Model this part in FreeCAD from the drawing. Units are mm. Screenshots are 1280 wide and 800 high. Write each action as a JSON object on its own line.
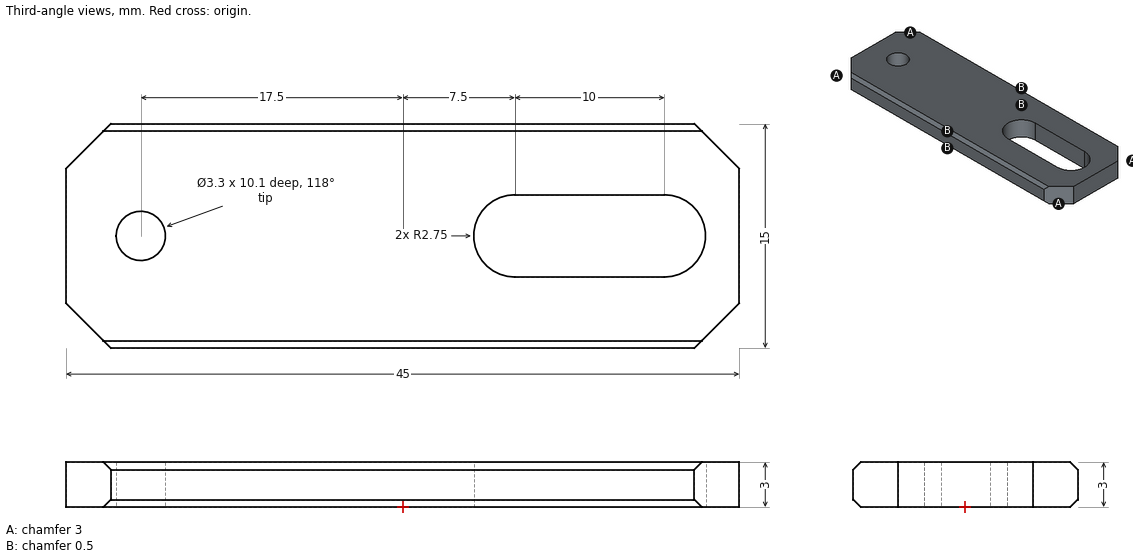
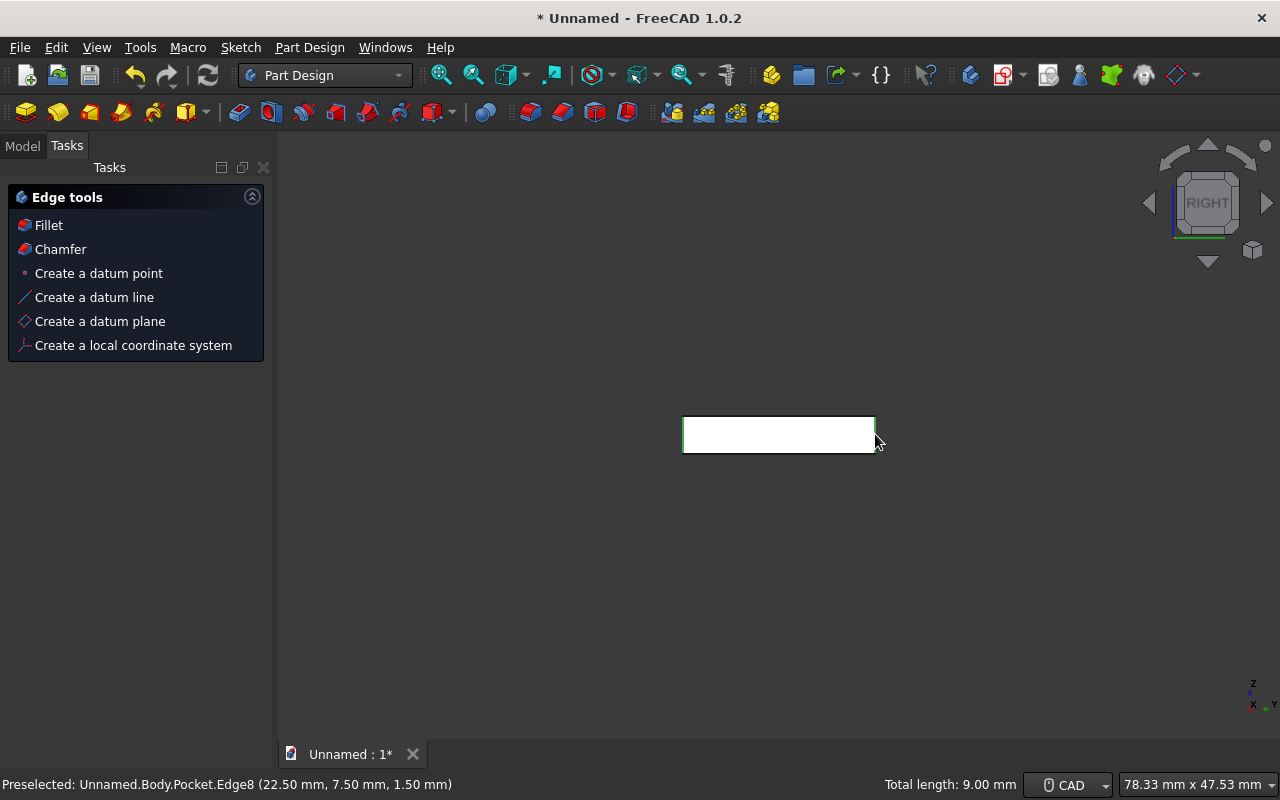
{"action": "key", "text": "5"}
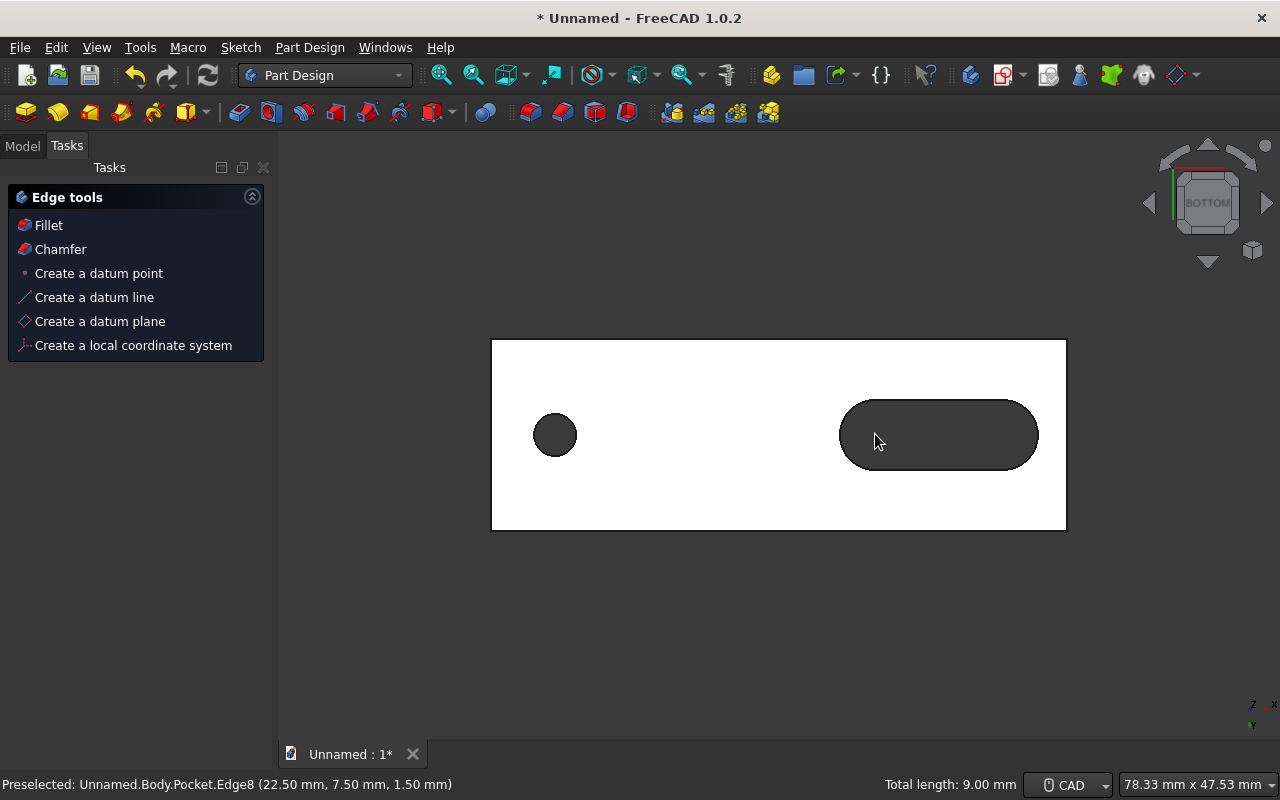
{"action": "key", "text": "4"}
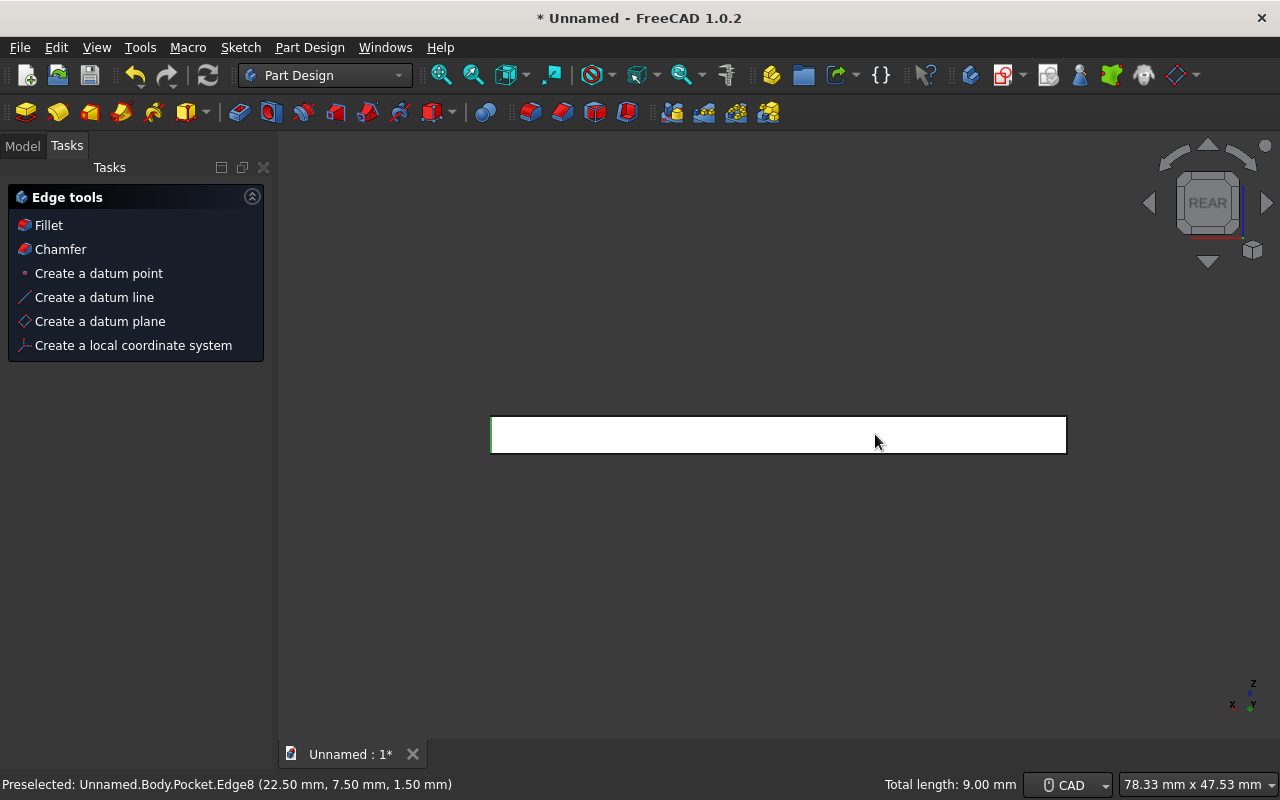
{"action": "left_click", "coordinate": [1067, 434], "text": "ctrl"}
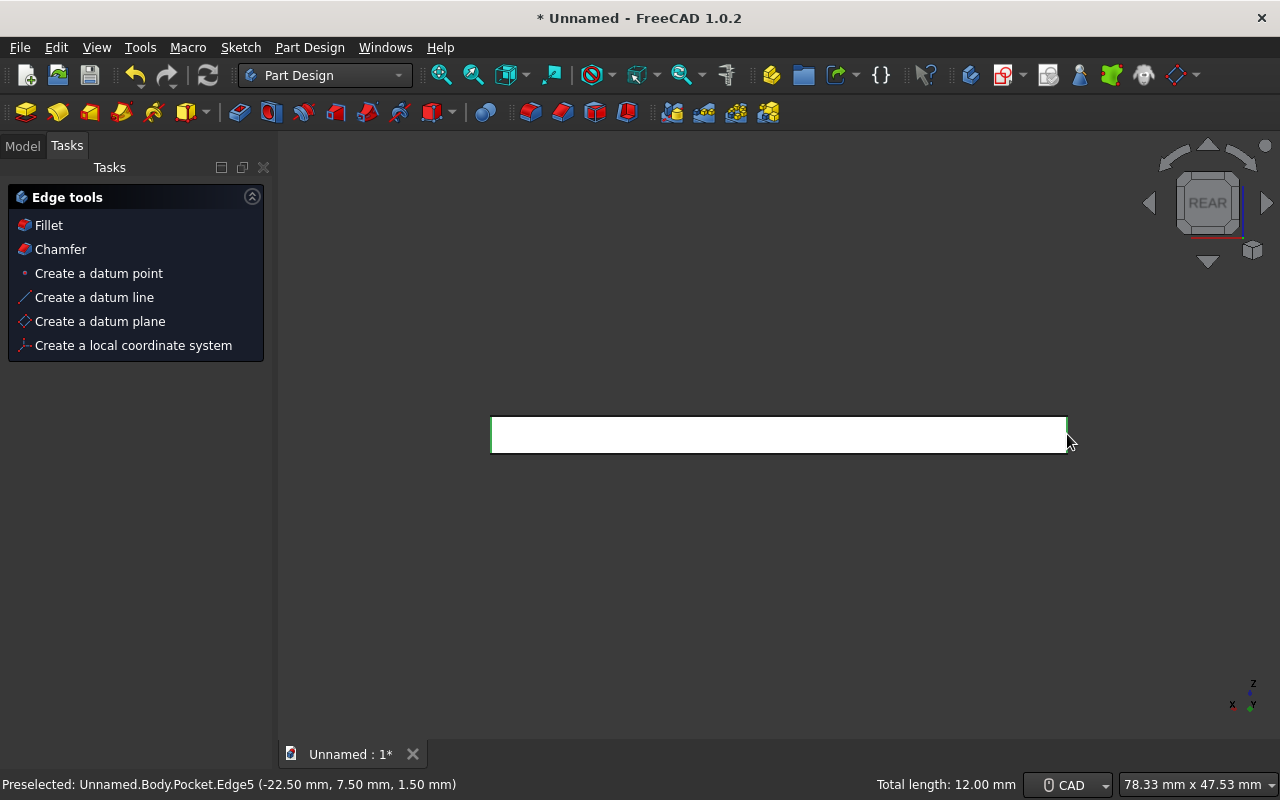
{"action": "left_click", "coordinate": [564, 112]}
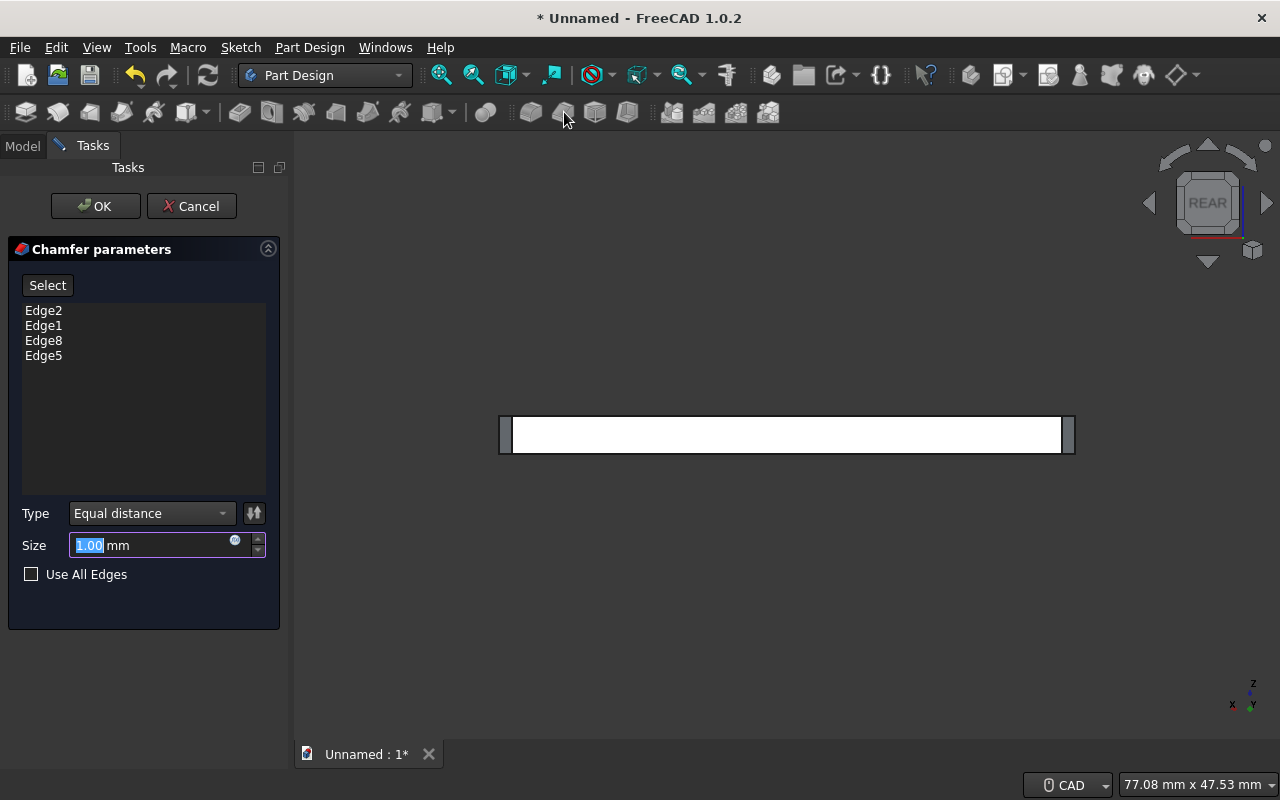
{"action": "type", "text": "3"}
{"action": "key", "text": "Tab"}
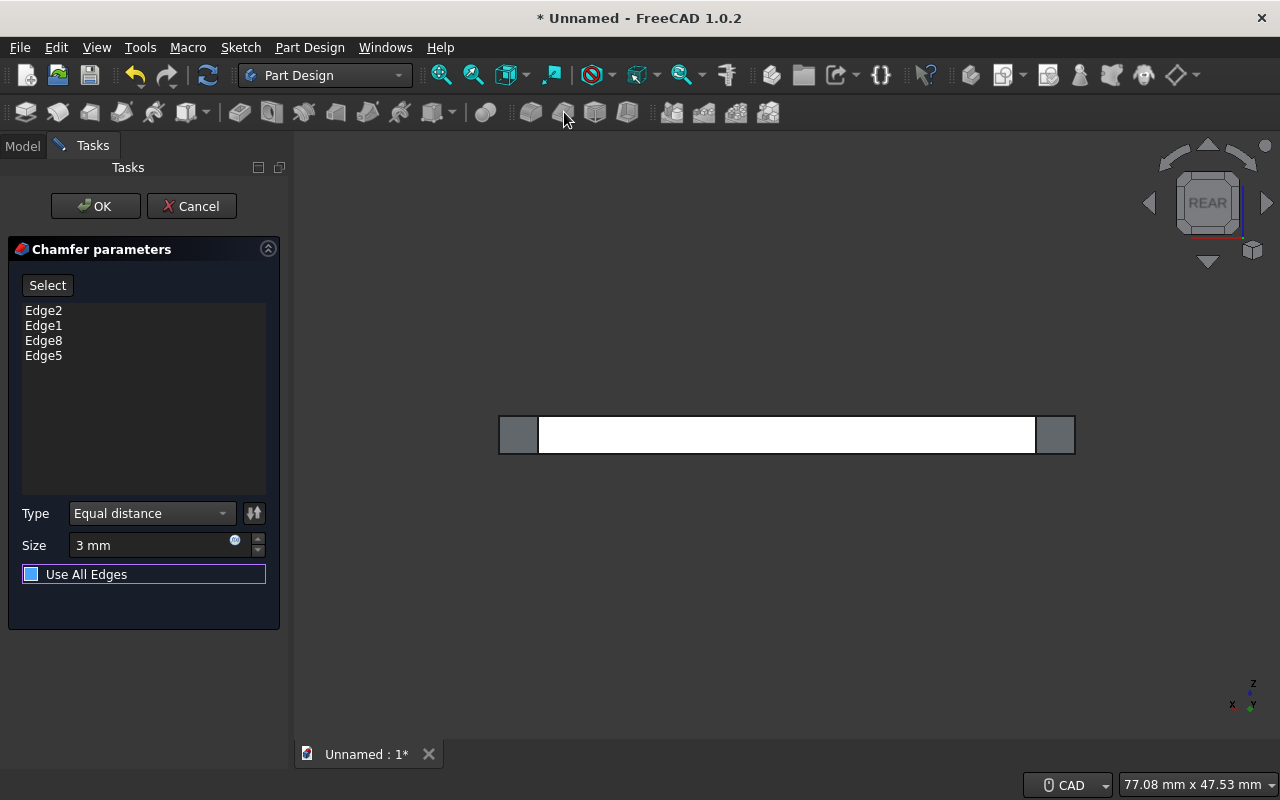
{"action": "left_click", "coordinate": [96, 206]}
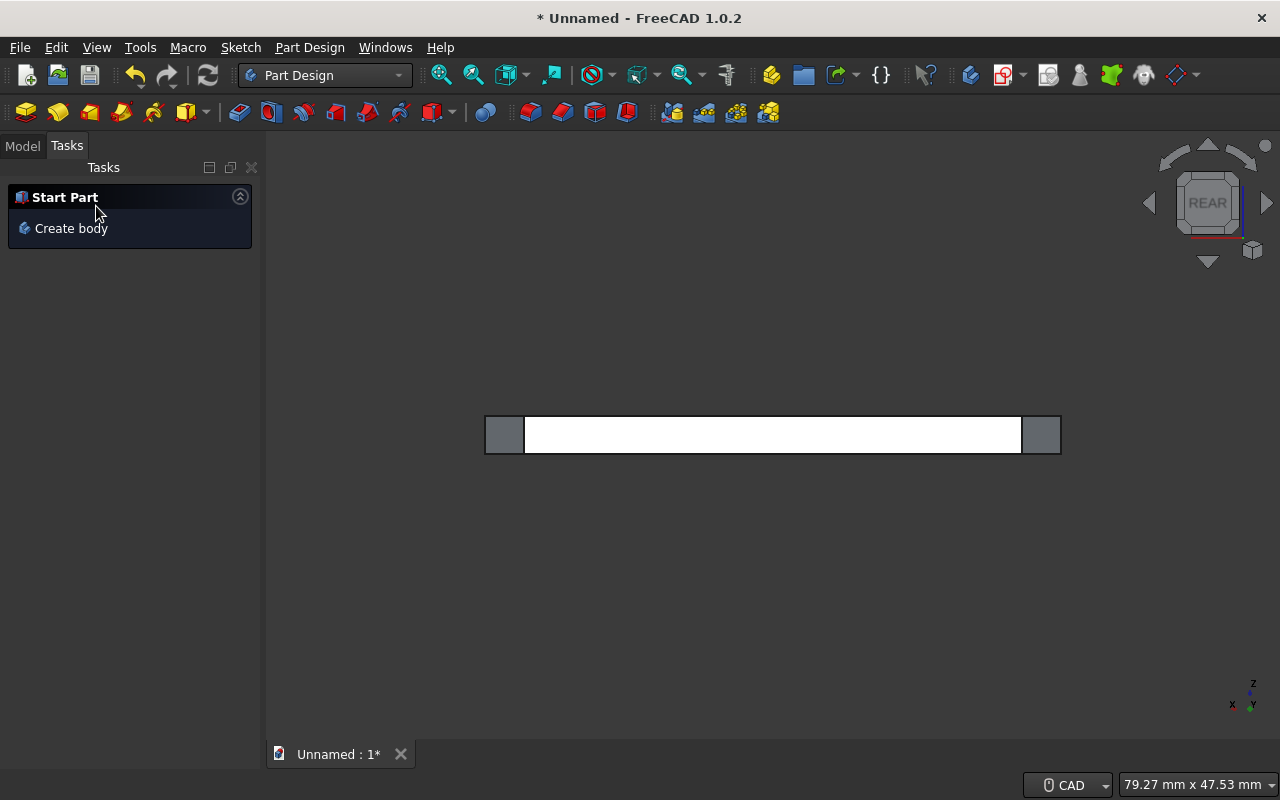
{"action": "left_click", "coordinate": [773, 453]}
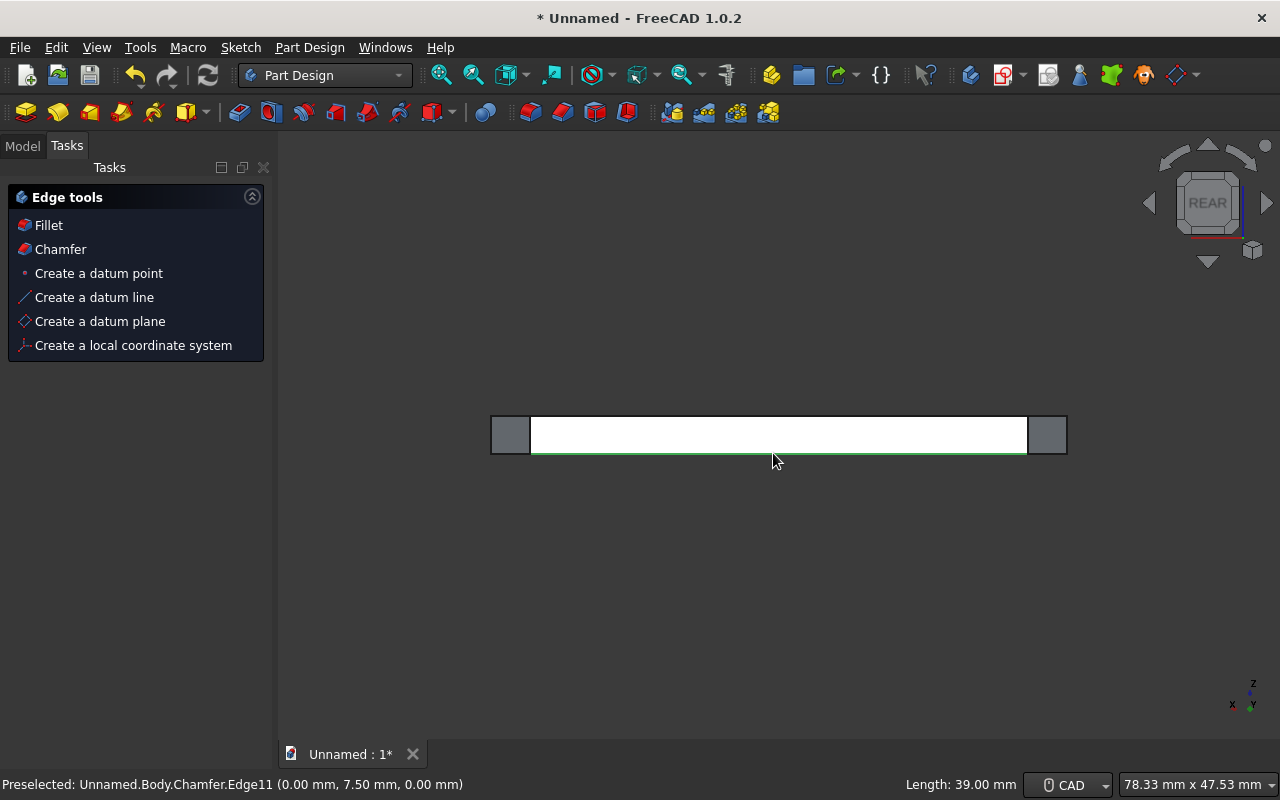
{"action": "left_click", "coordinate": [779, 415], "text": "ctrl"}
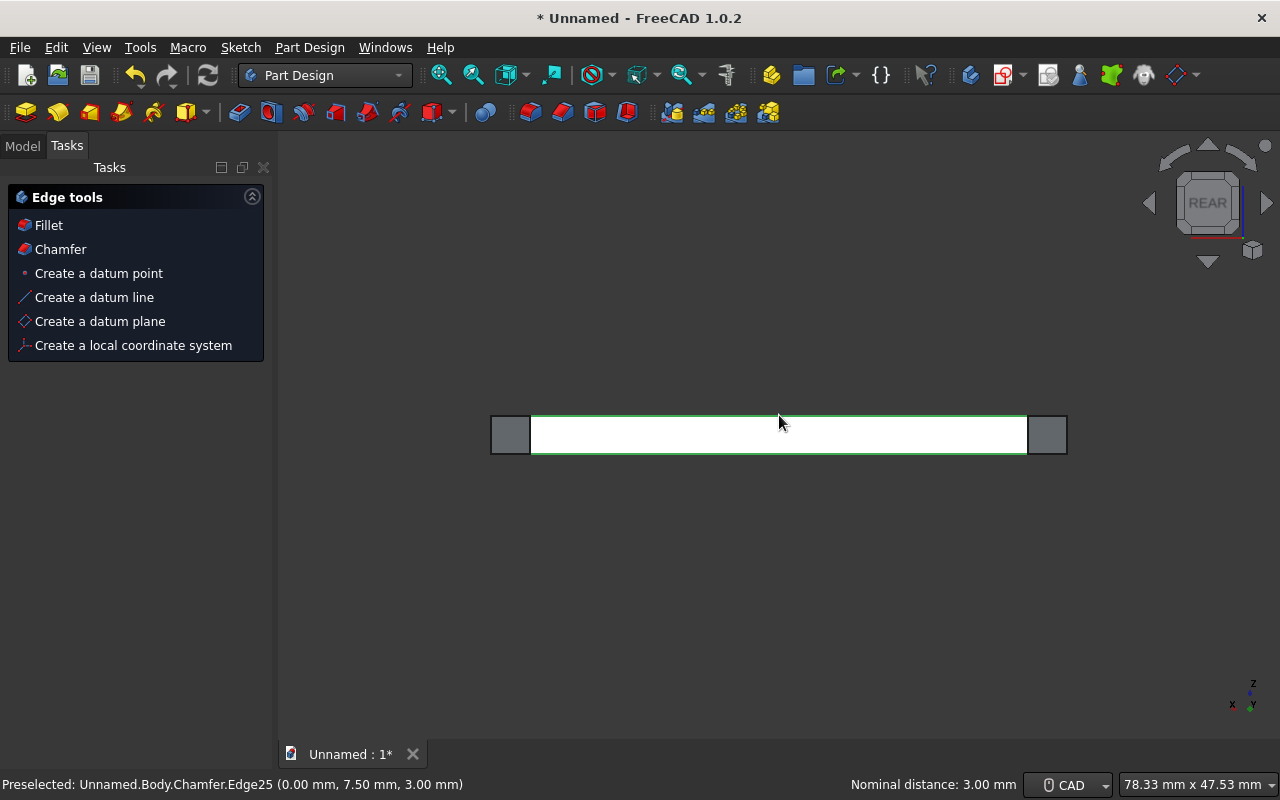
{"action": "key", "text": "0"}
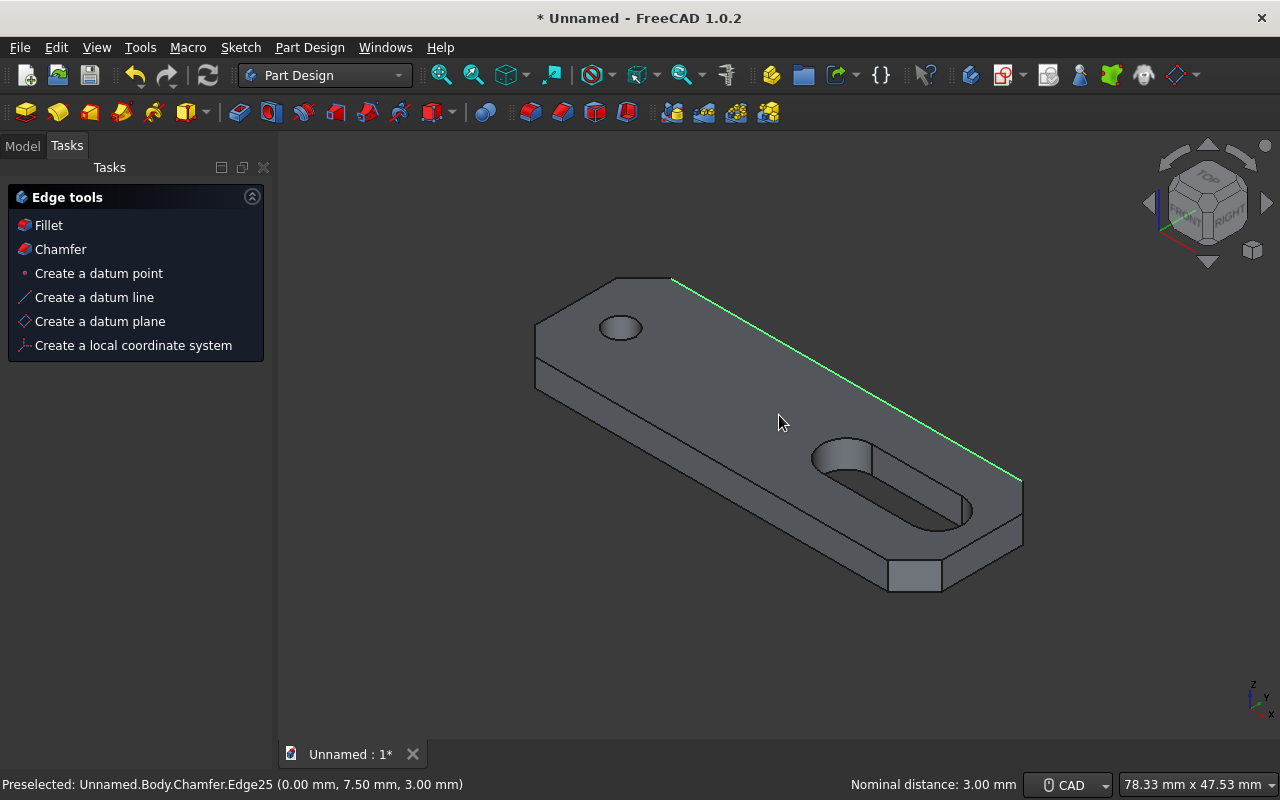
{"action": "left_click", "coordinate": [711, 458], "text": "ctrl"}